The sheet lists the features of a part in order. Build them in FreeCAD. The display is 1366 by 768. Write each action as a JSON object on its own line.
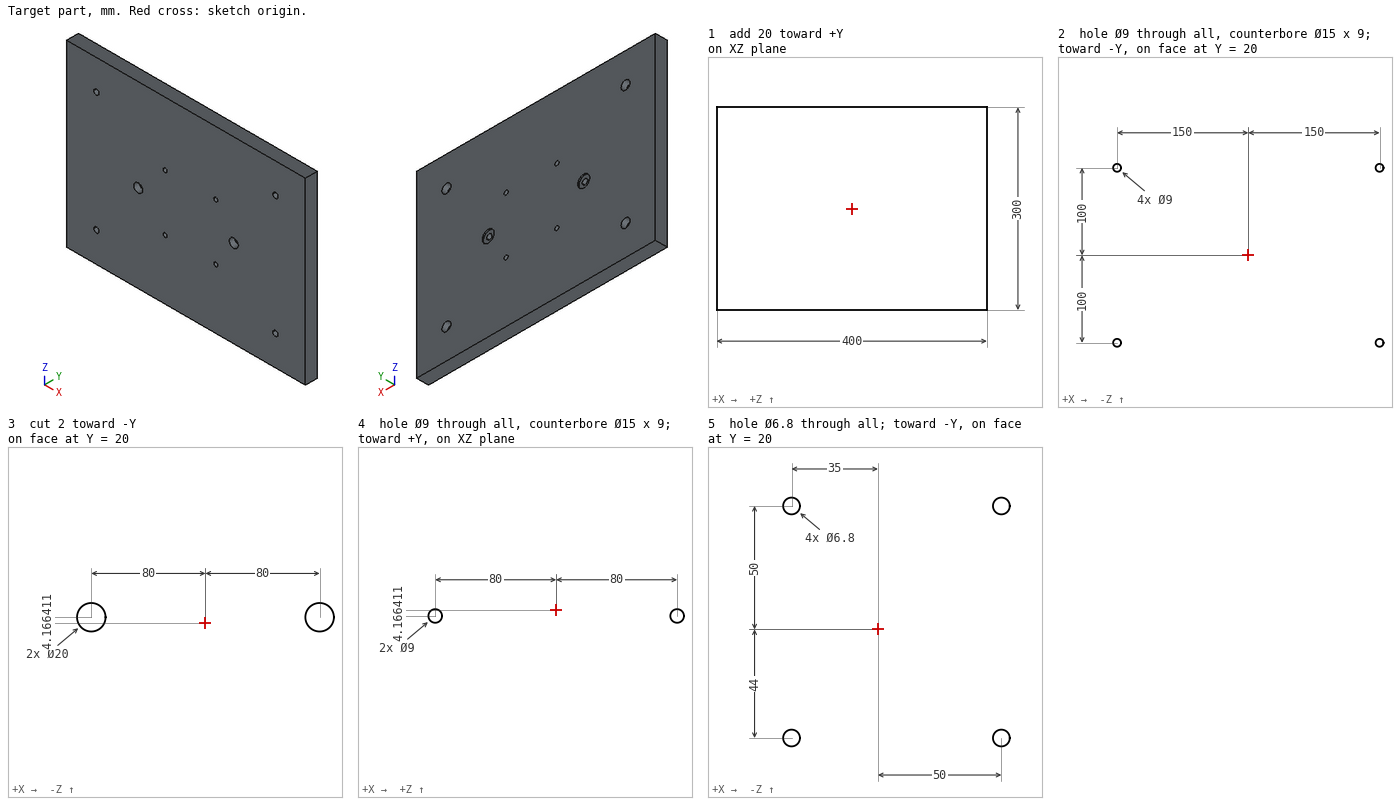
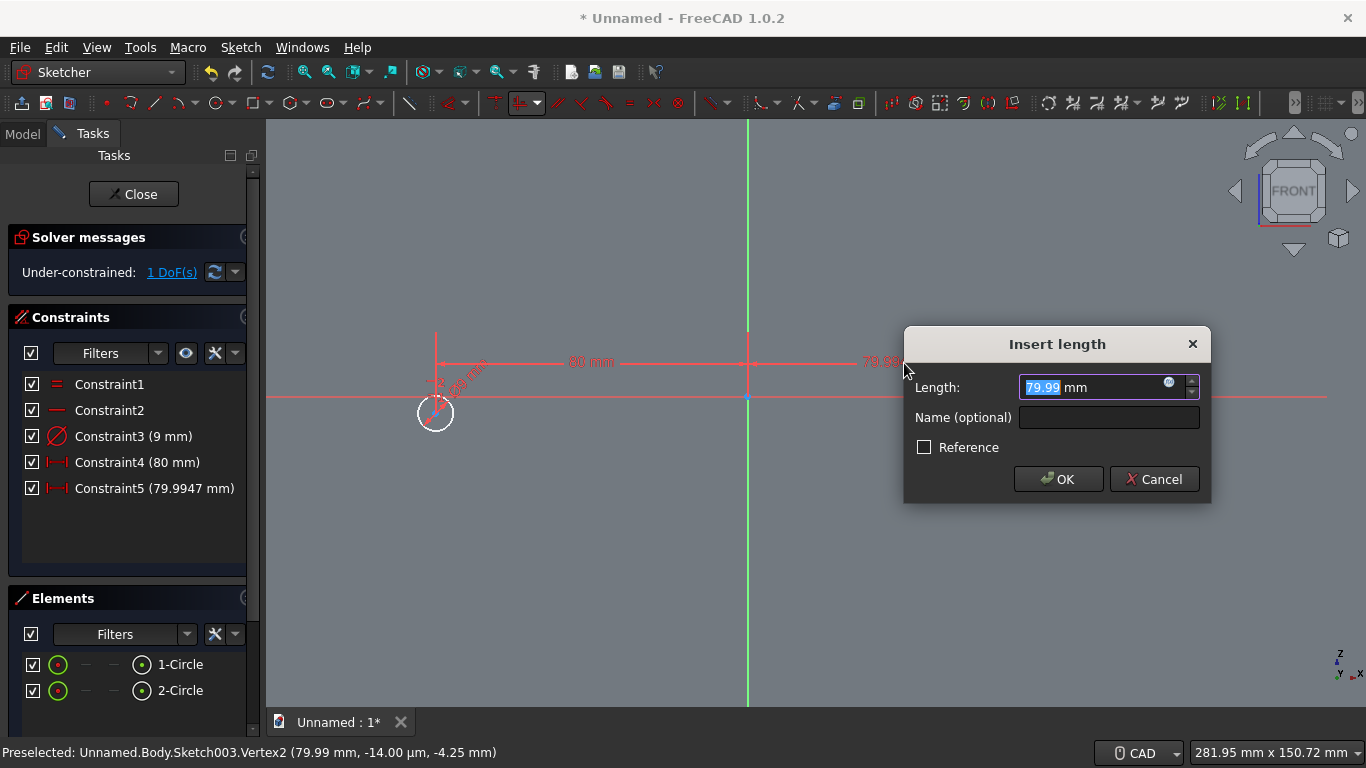
{"action": "type", "text": "80"}
{"action": "key", "text": "Return"}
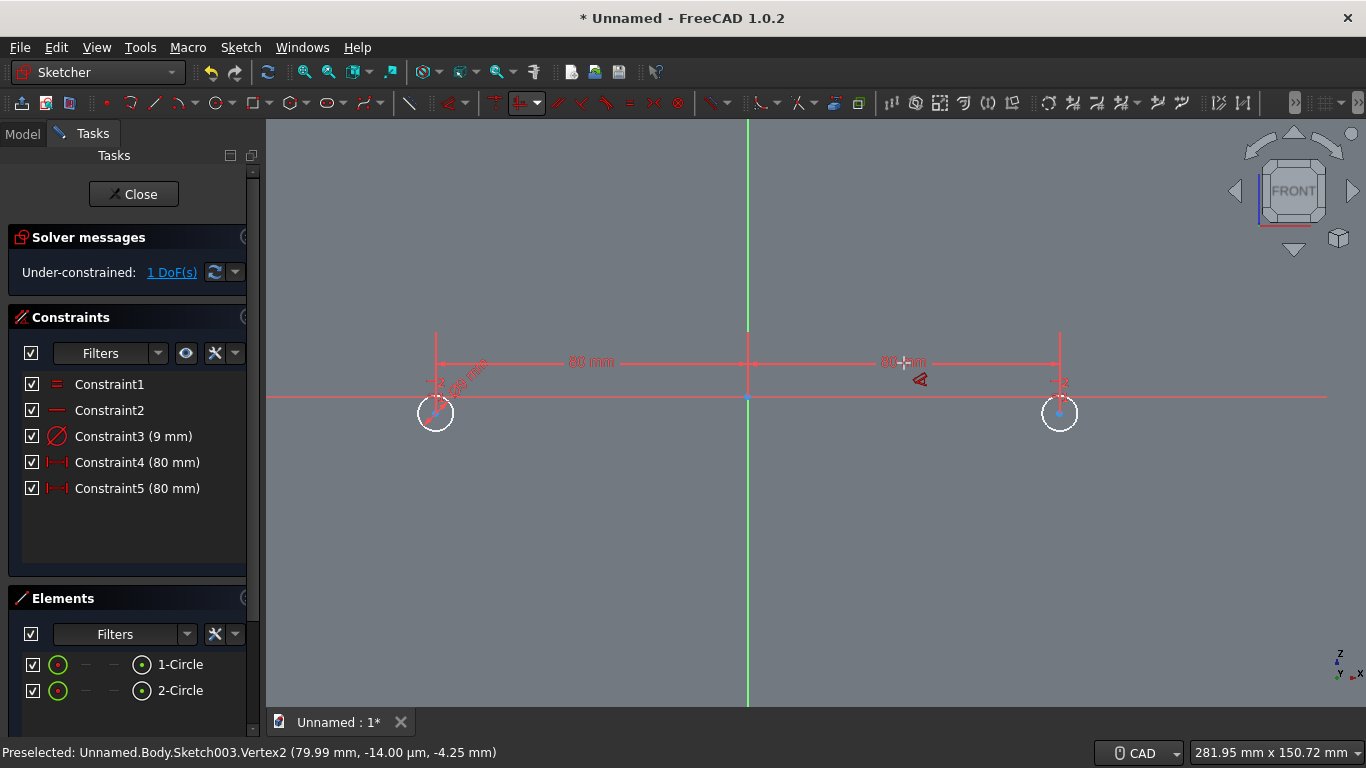
{"action": "scroll", "coordinate": [436, 413], "scroll_direction": "up", "scroll_amount": 5}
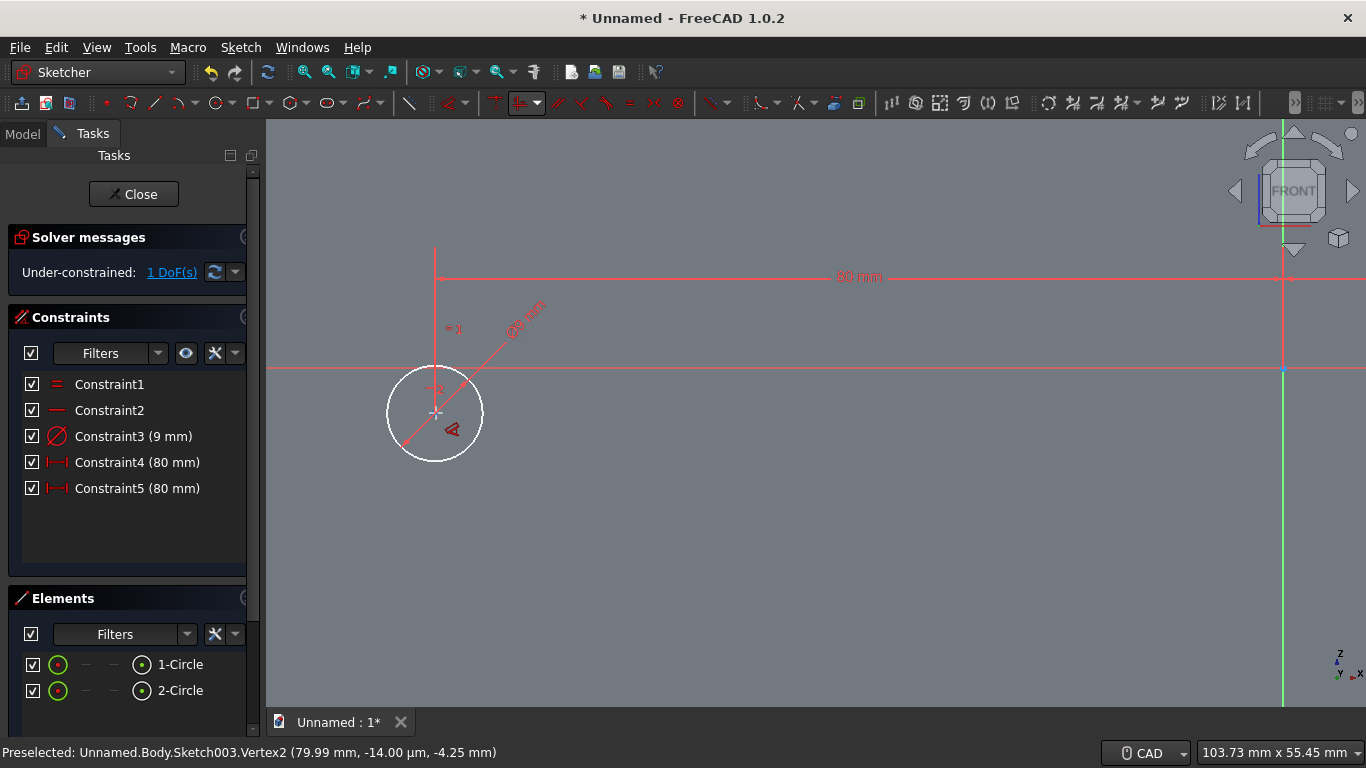
{"action": "left_click", "coordinate": [435, 413]}
{"action": "left_click", "coordinate": [401, 407]}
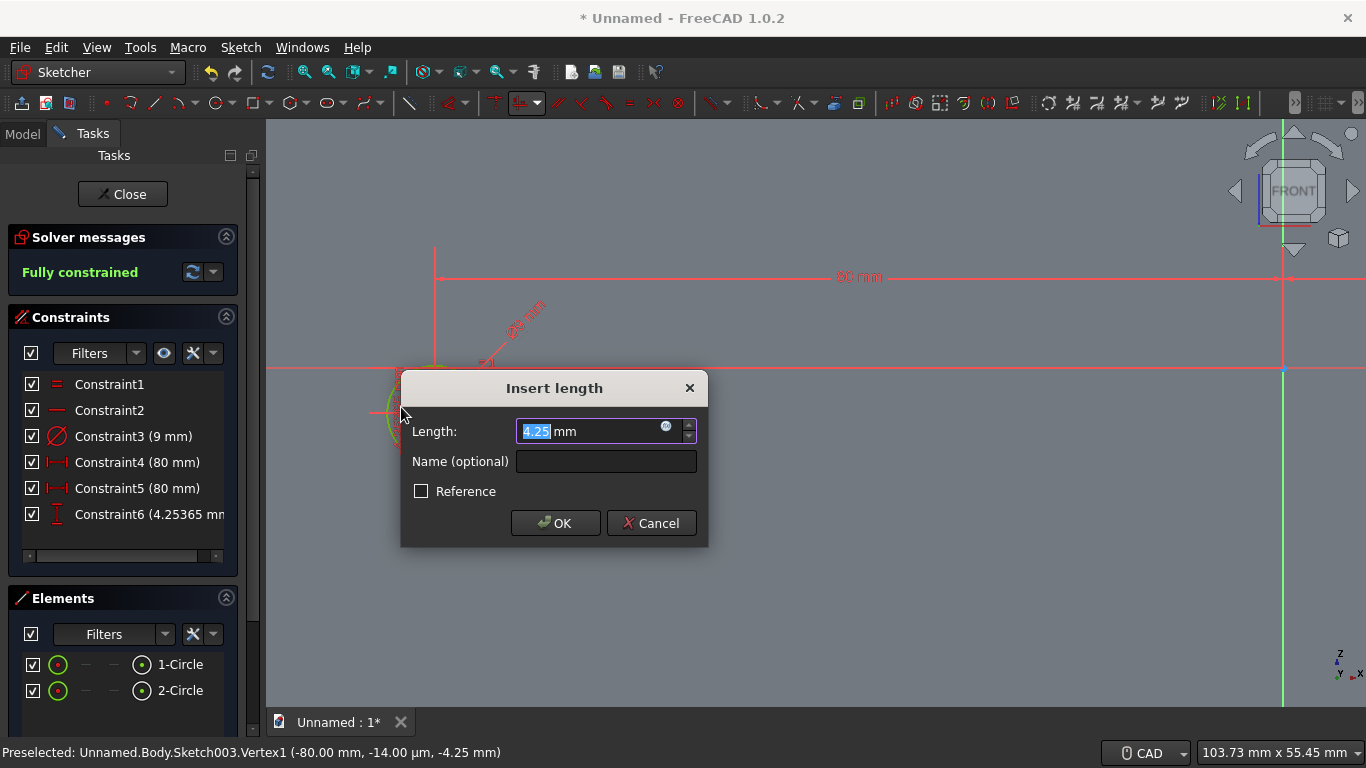
{"action": "type", "text": "4.166411"}
{"action": "key", "text": "Return"}
{"action": "key", "text": "Escape"}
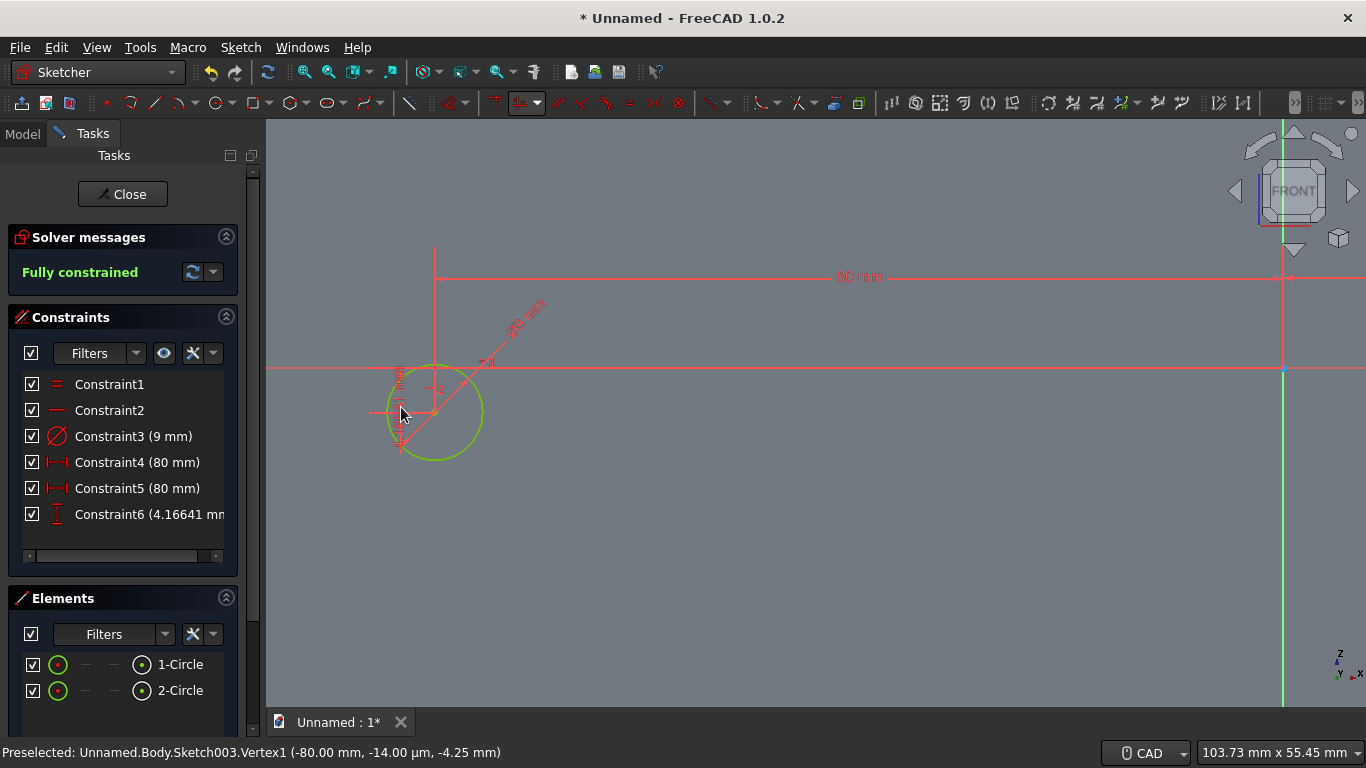
{"action": "left_click", "coordinate": [123, 194]}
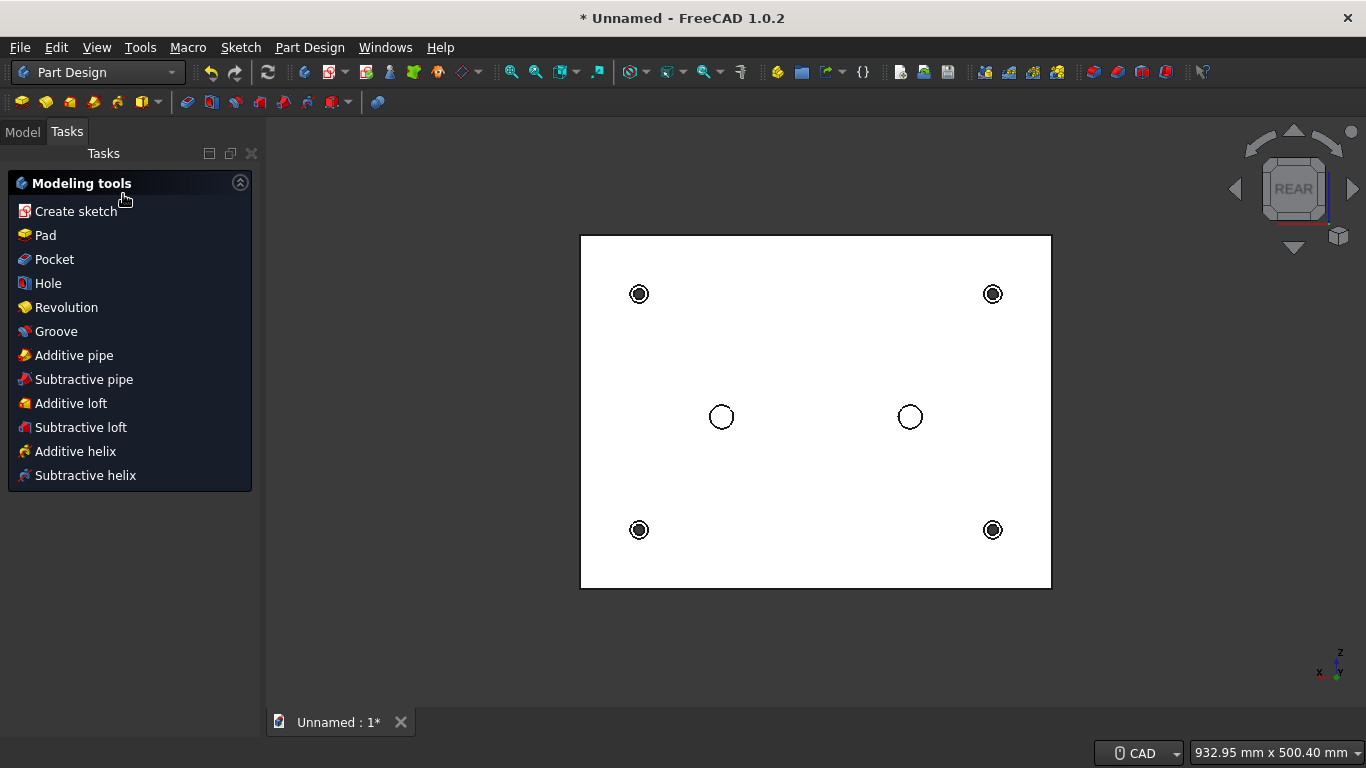
{"action": "left_click", "coordinate": [212, 102]}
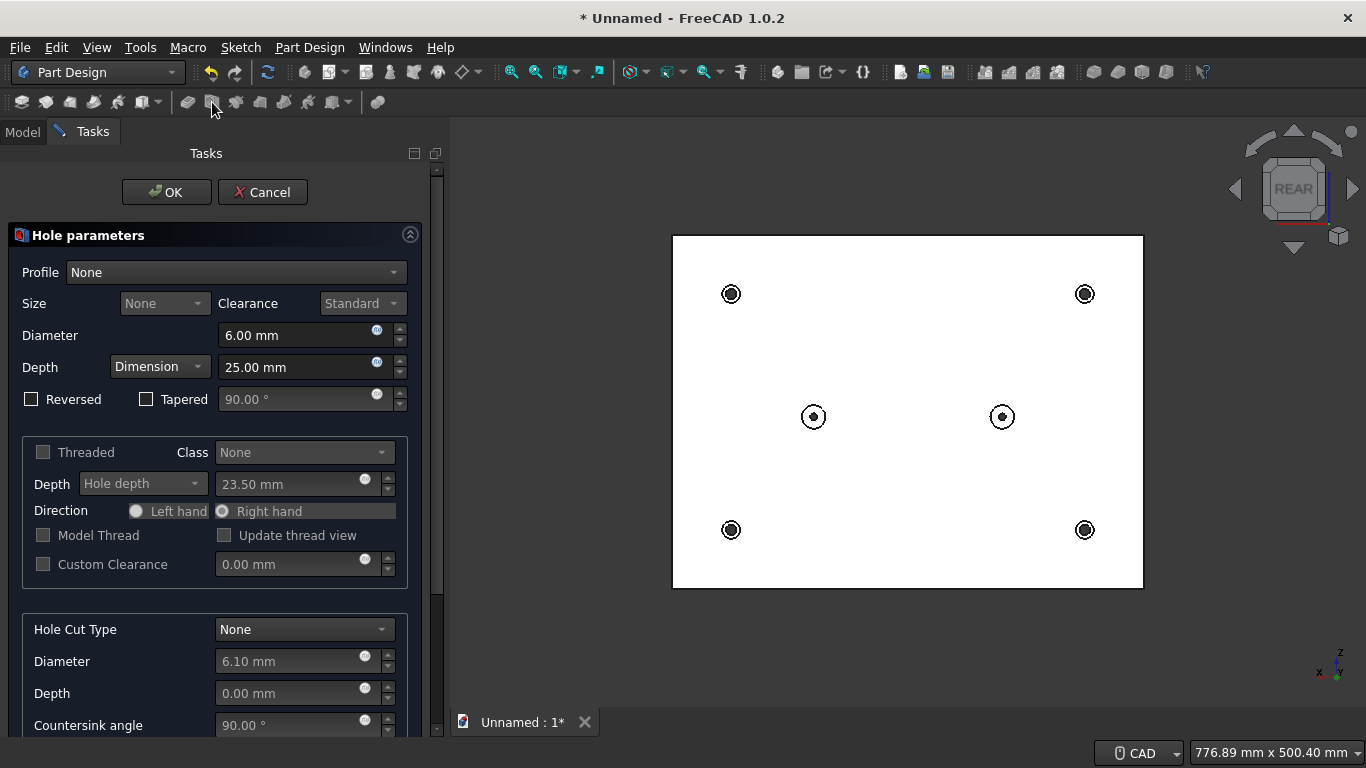
{"action": "triple_click", "coordinate": [305, 335]}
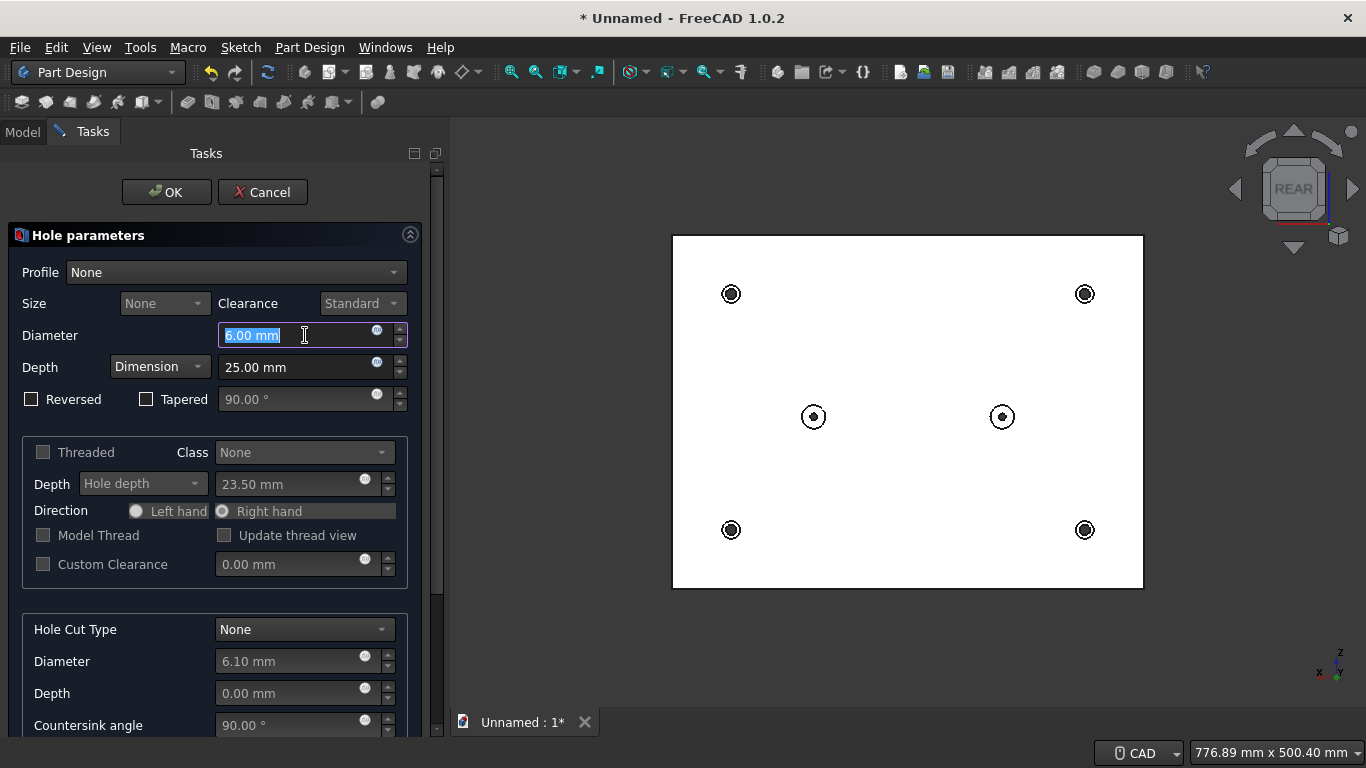
{"action": "type", "text": "9"}
{"action": "key", "text": "Tab"}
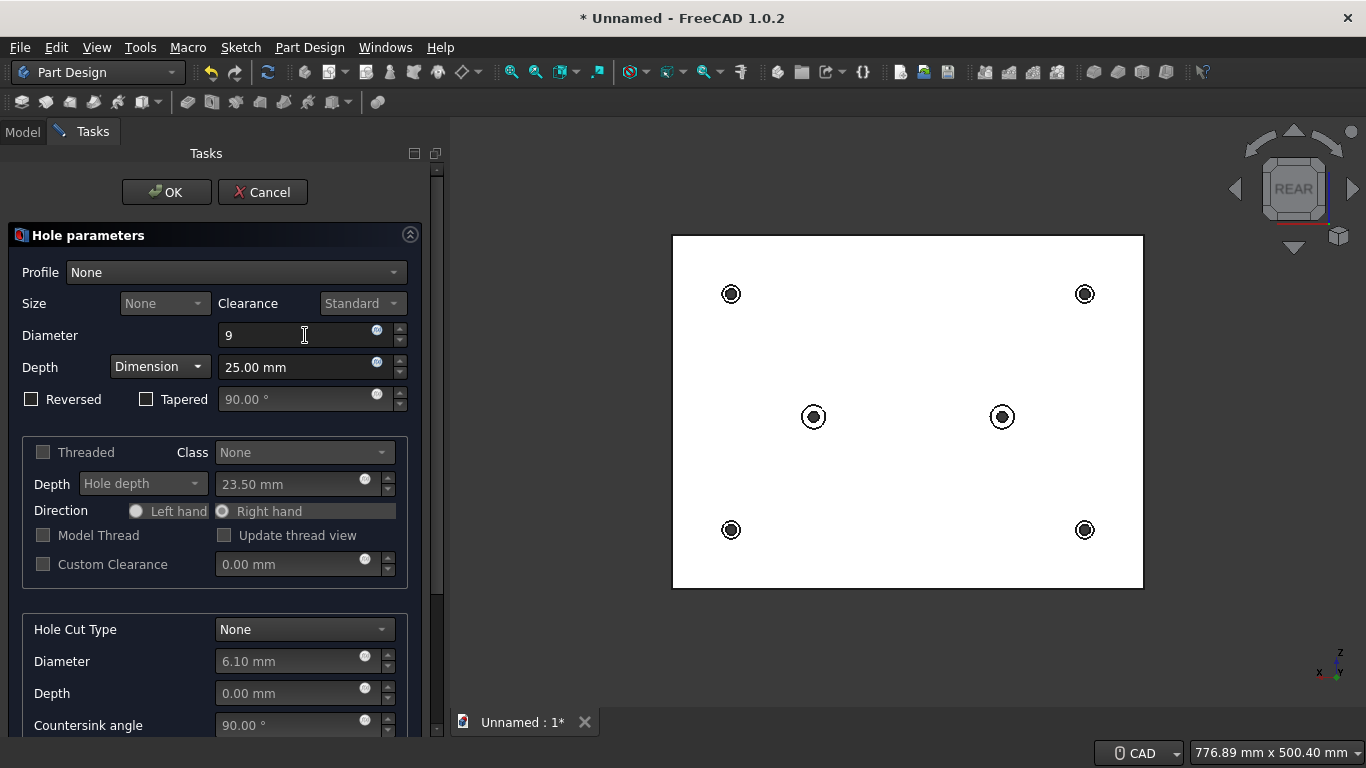
{"action": "left_click", "coordinate": [161, 366]}